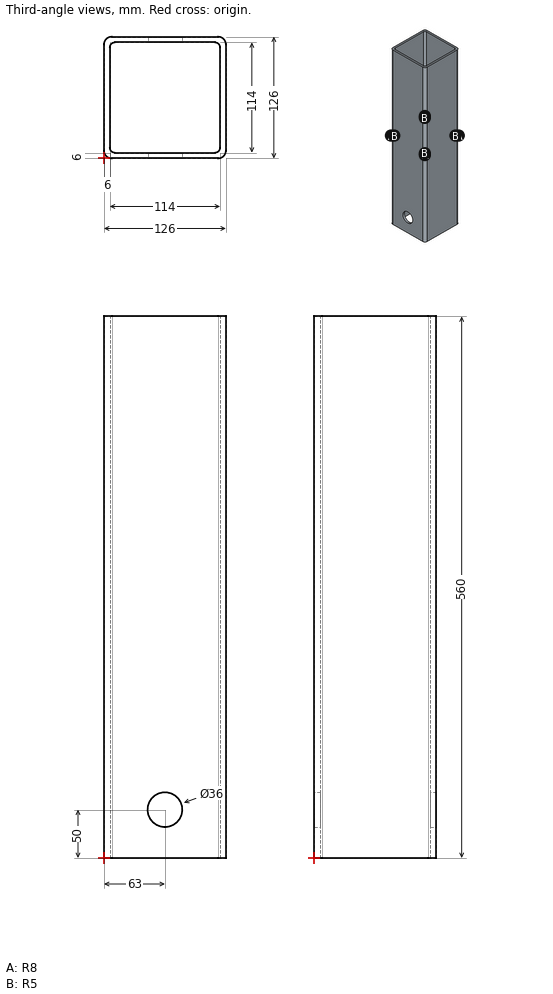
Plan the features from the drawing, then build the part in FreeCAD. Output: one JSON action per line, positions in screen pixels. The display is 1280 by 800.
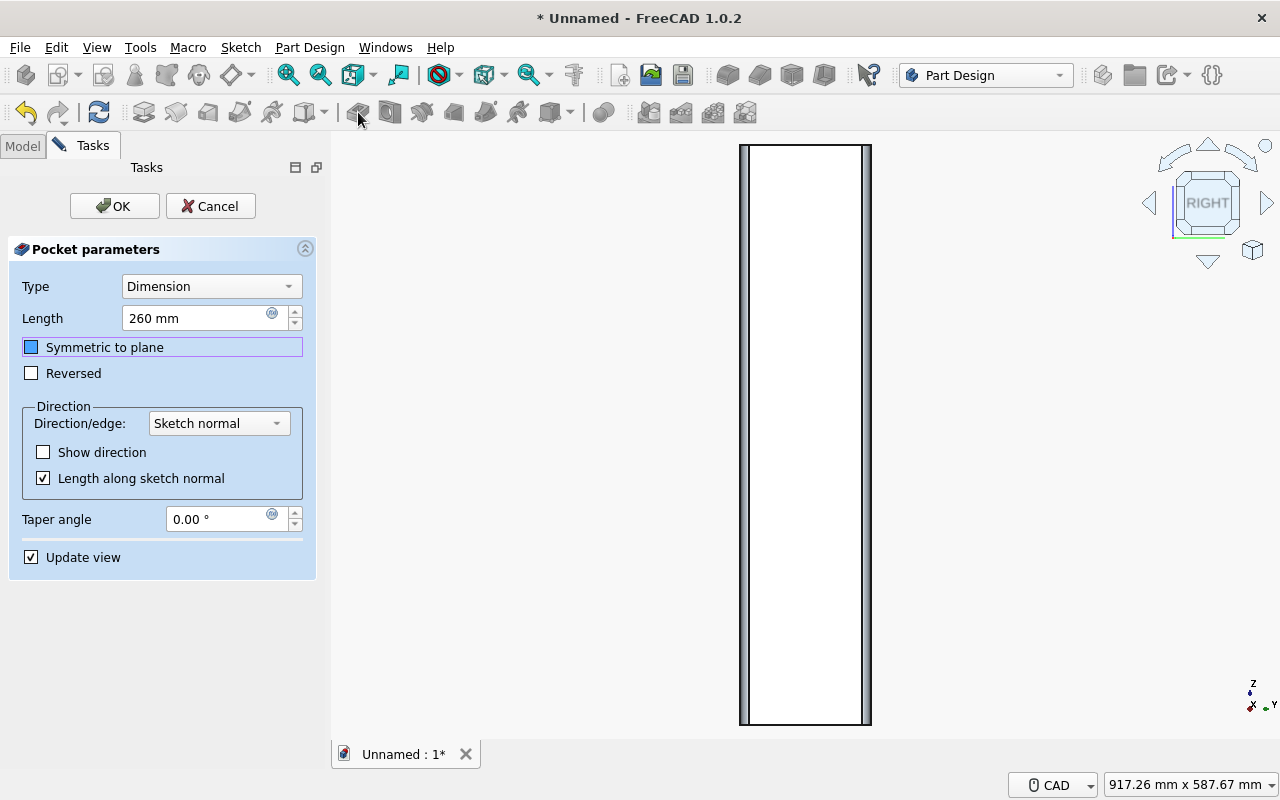
{"action": "left_click", "coordinate": [115, 206]}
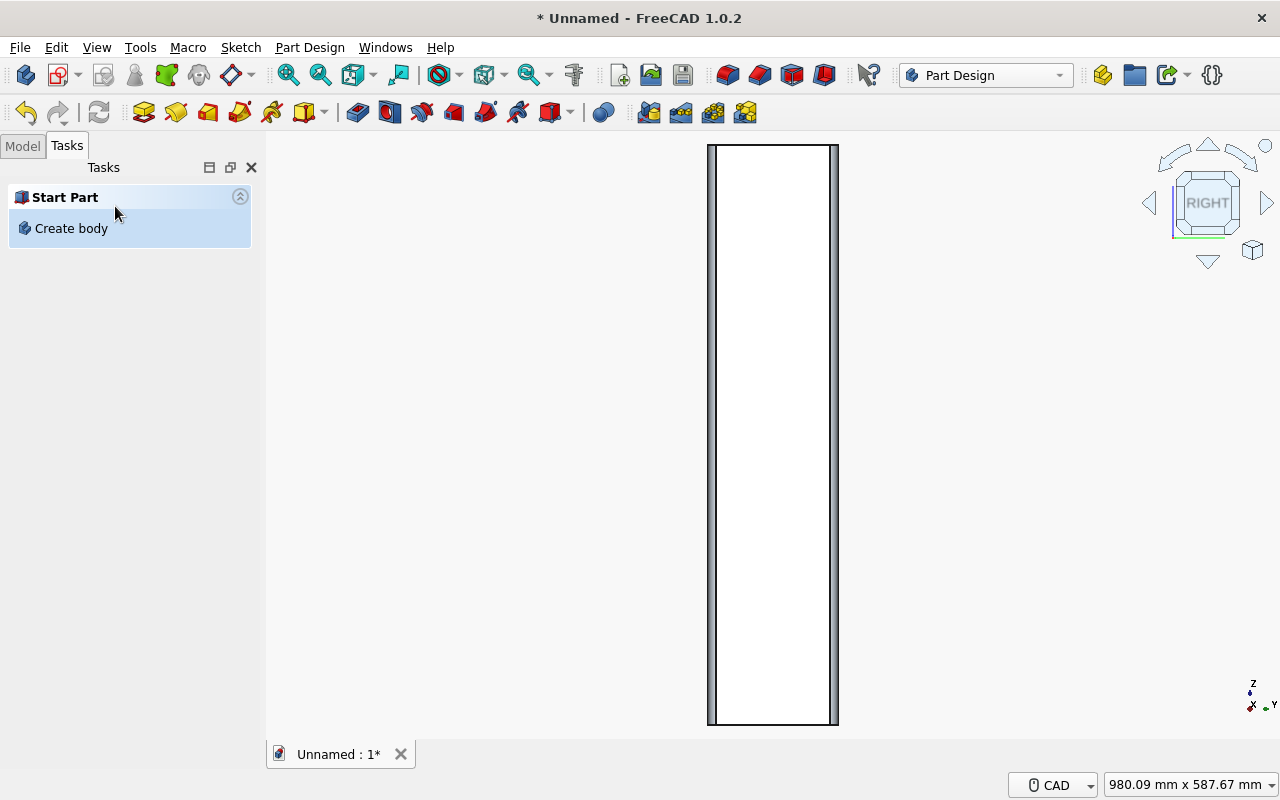
{"action": "key", "text": "0"}